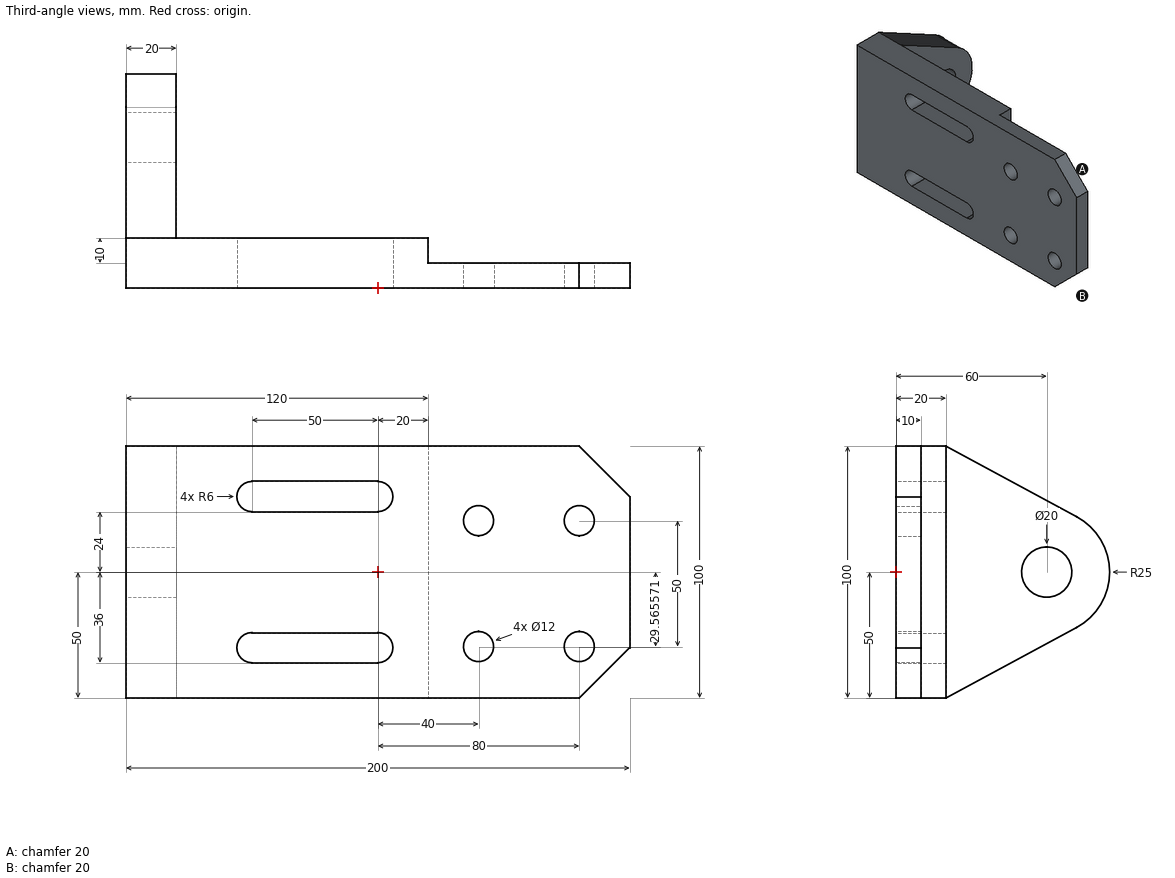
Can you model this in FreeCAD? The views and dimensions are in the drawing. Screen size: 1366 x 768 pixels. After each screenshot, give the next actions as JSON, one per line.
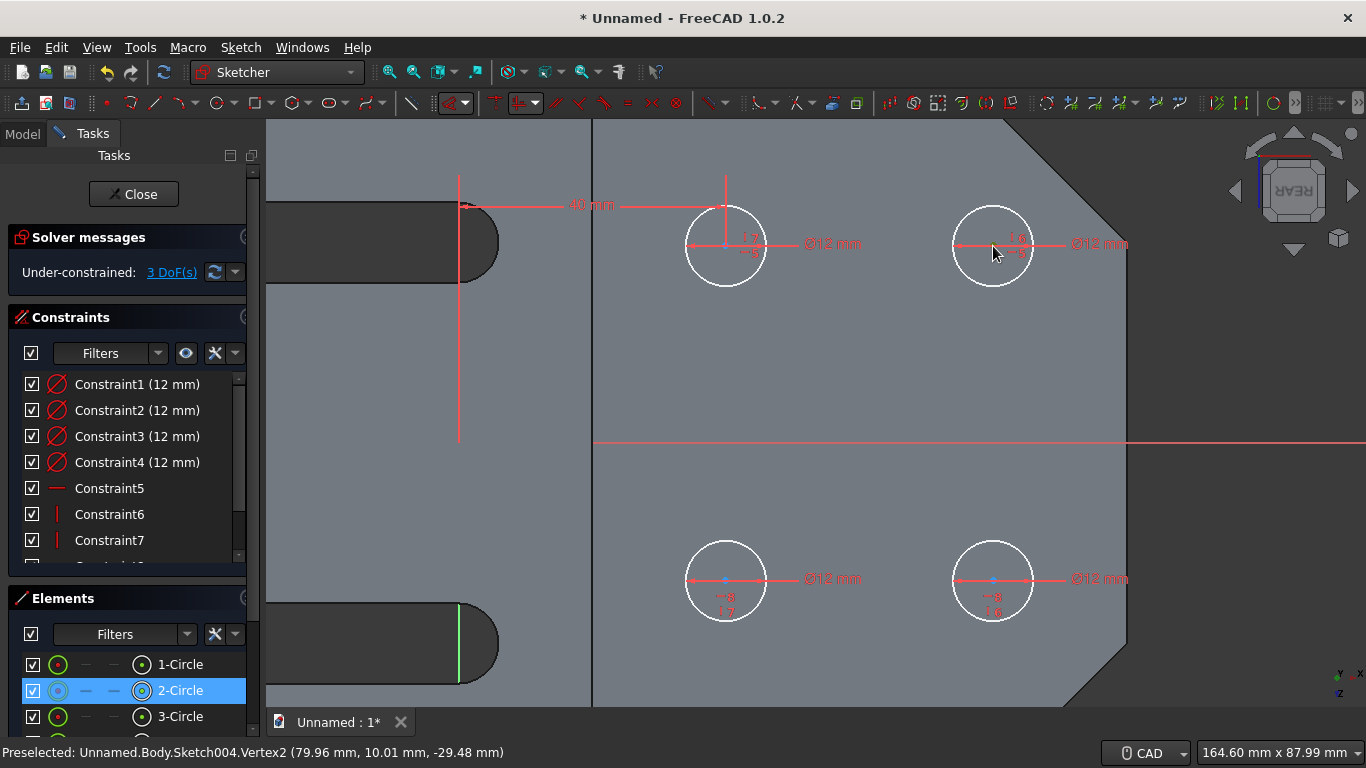
{"action": "left_click", "coordinate": [468, 104]}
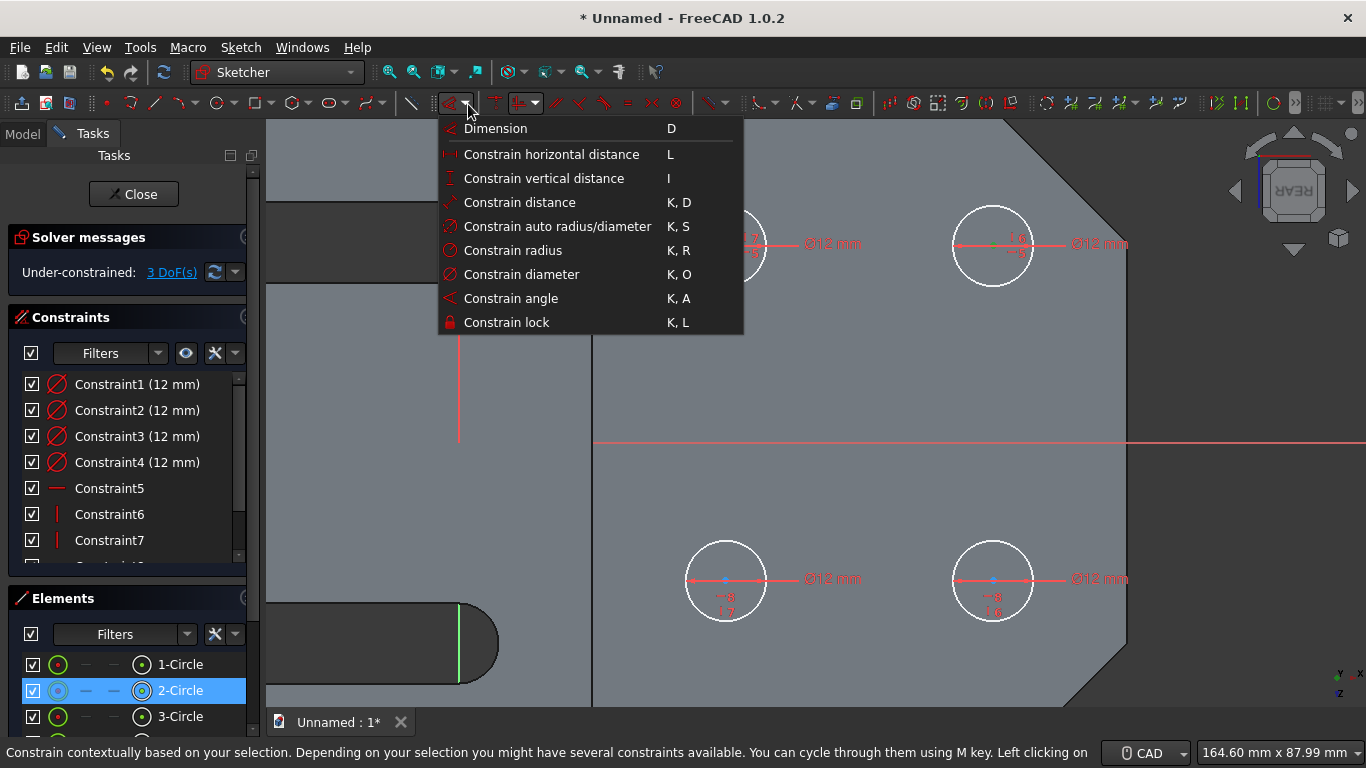
{"action": "left_click", "coordinate": [591, 154]}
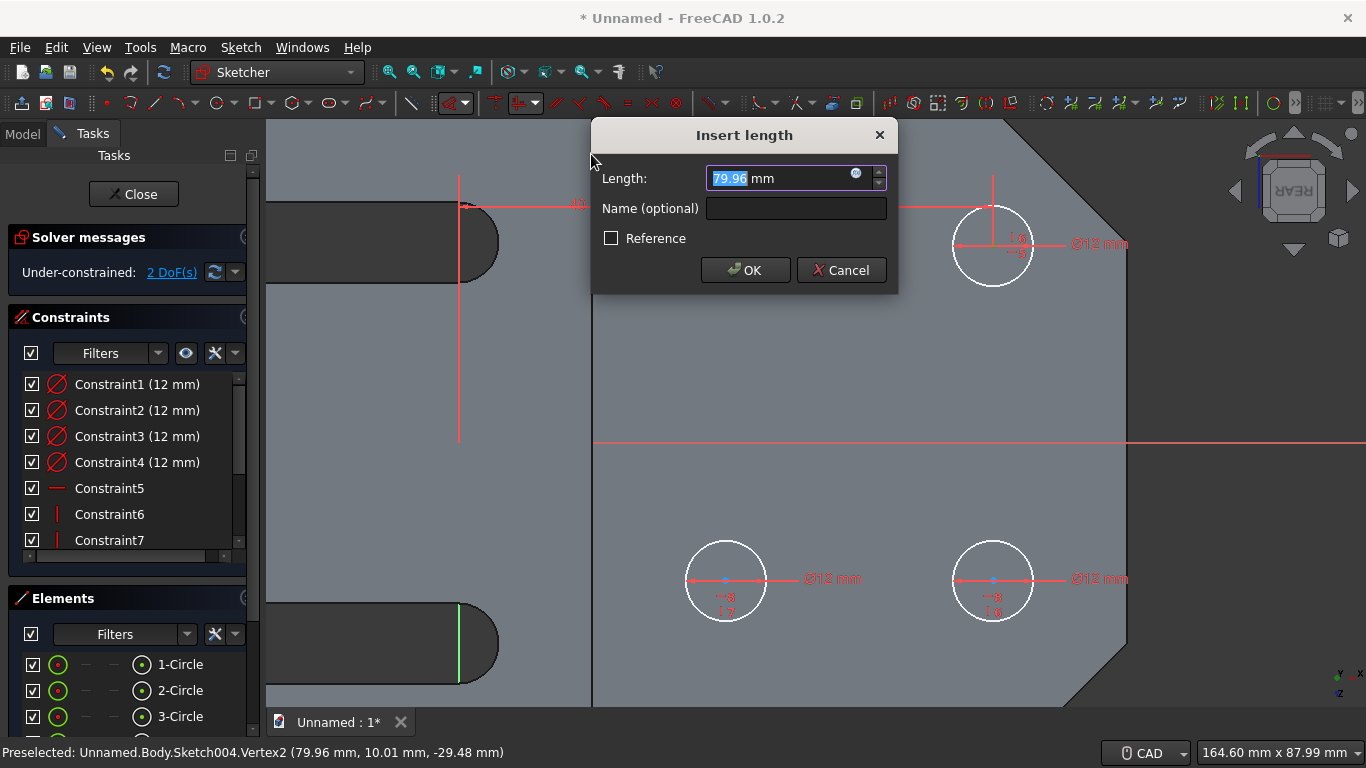
{"action": "type", "text": "80"}
{"action": "key", "text": "Return"}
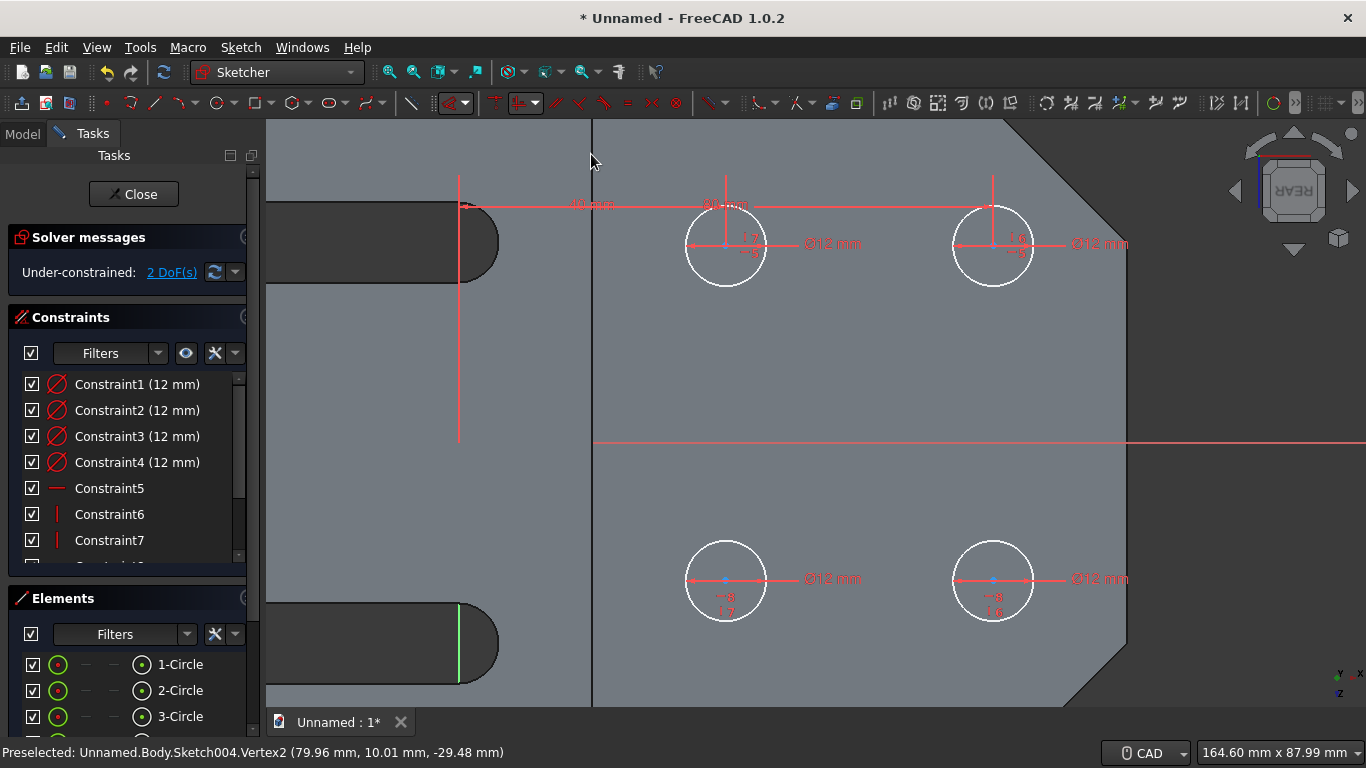
{"action": "left_click", "coordinate": [993, 246]}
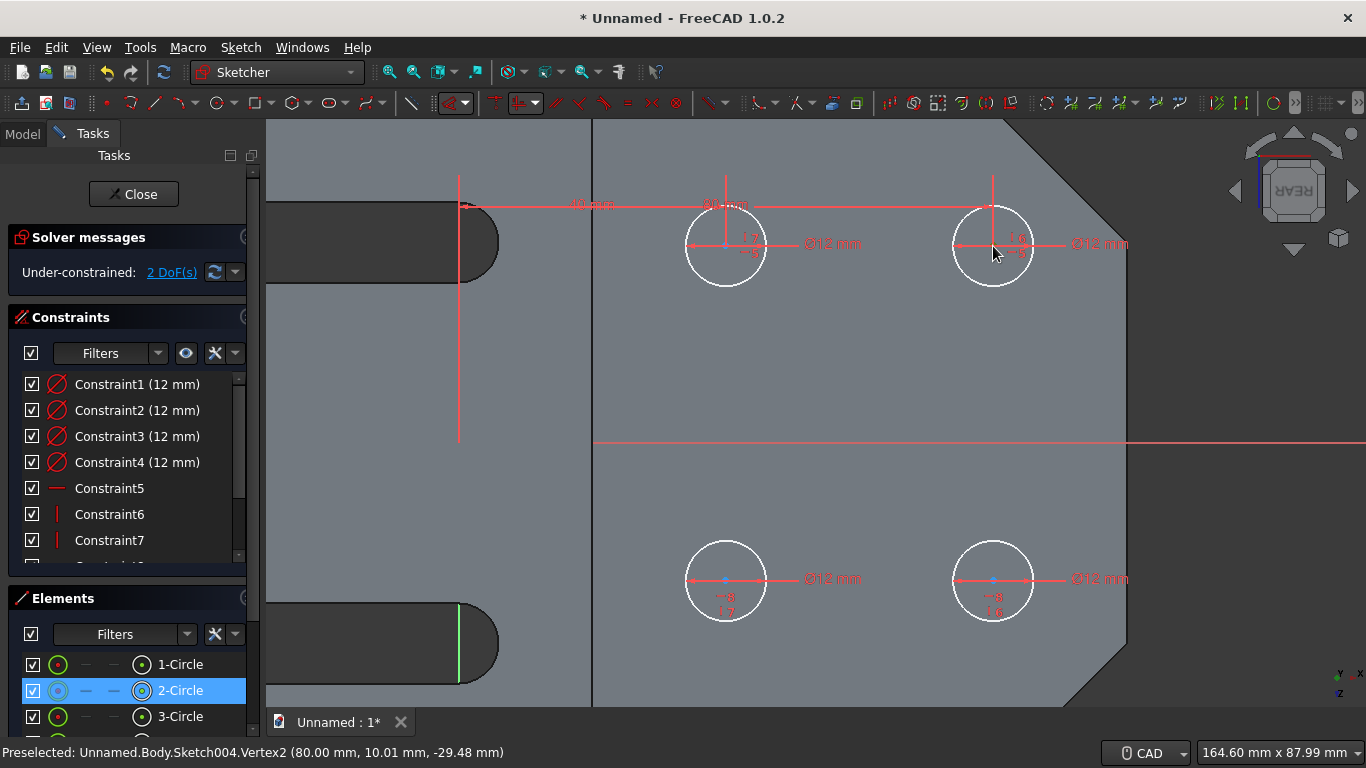
{"action": "left_click", "coordinate": [993, 581]}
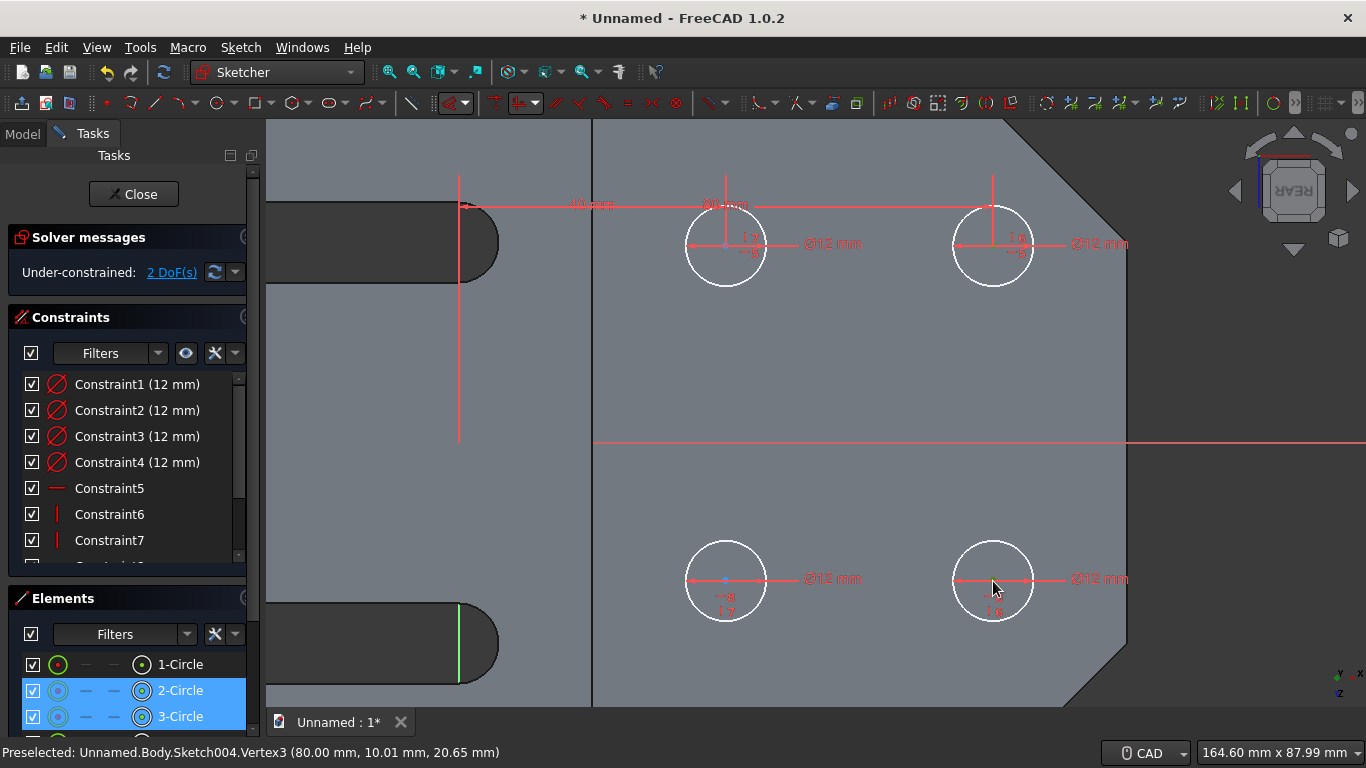
{"action": "left_click", "coordinate": [468, 104]}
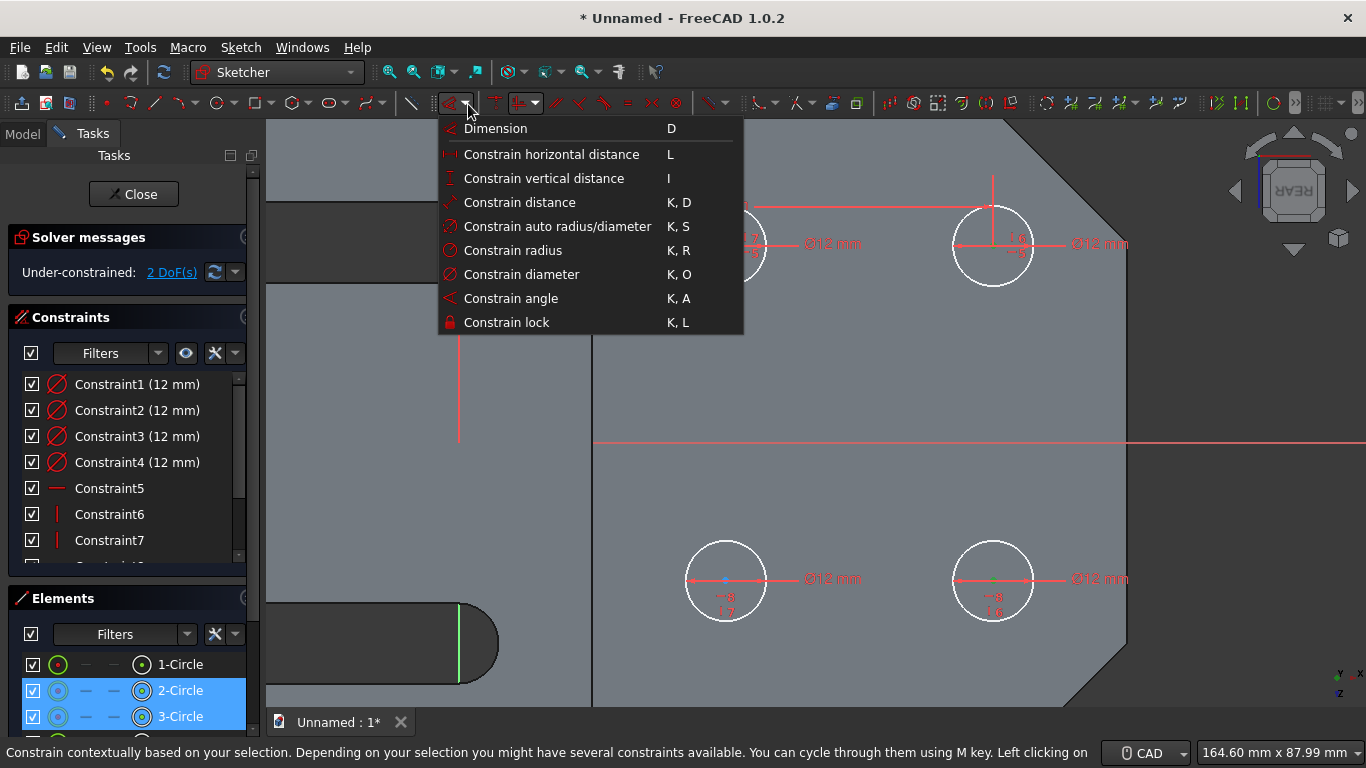
{"action": "left_click", "coordinate": [591, 178]}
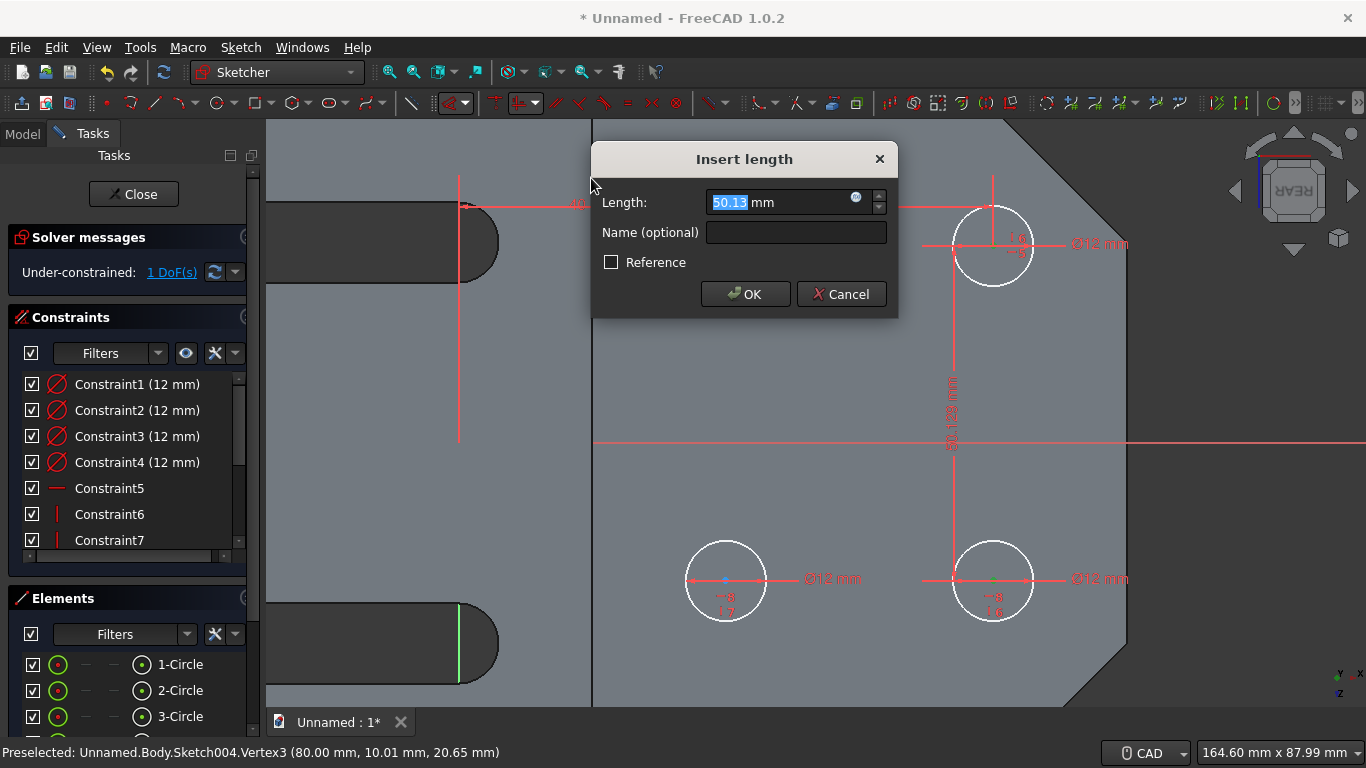
{"action": "type", "text": "50"}
{"action": "key", "text": "Return"}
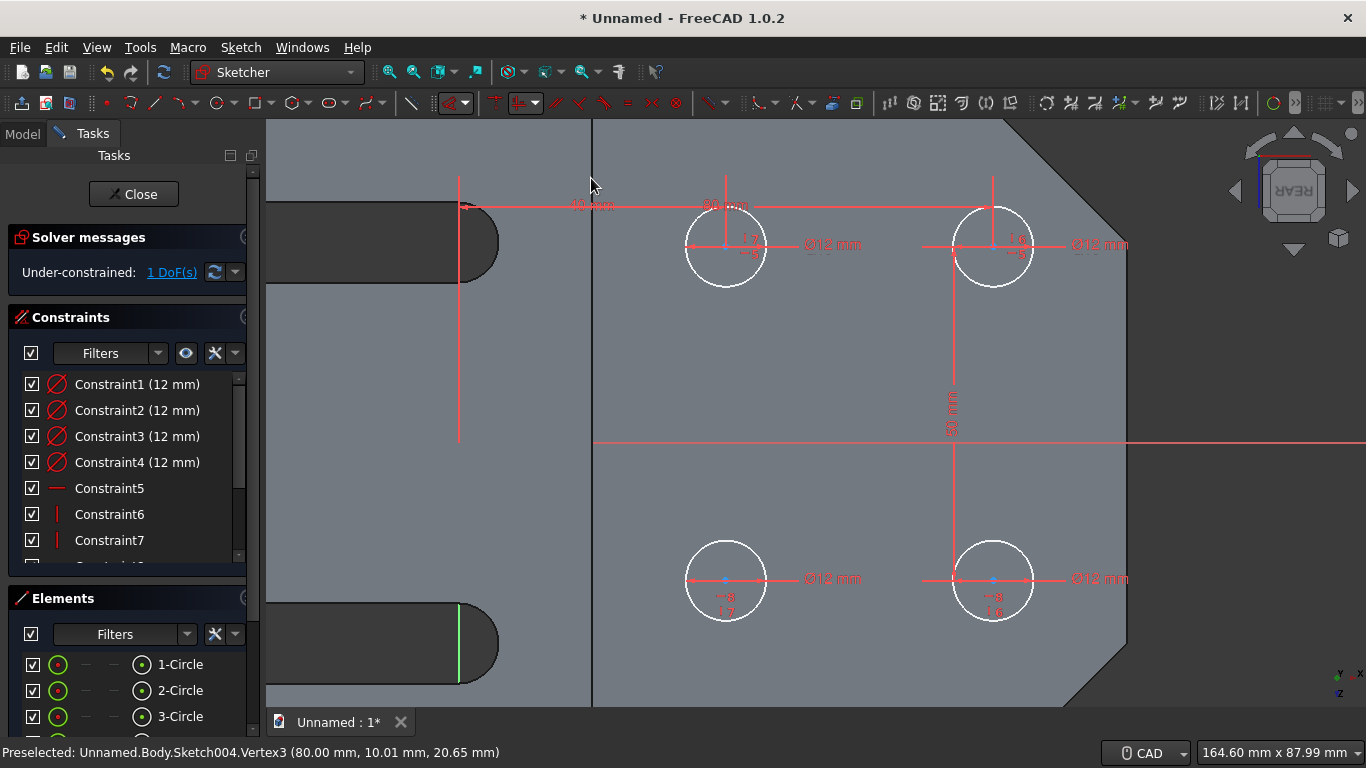
{"action": "left_click", "coordinate": [726, 247]}